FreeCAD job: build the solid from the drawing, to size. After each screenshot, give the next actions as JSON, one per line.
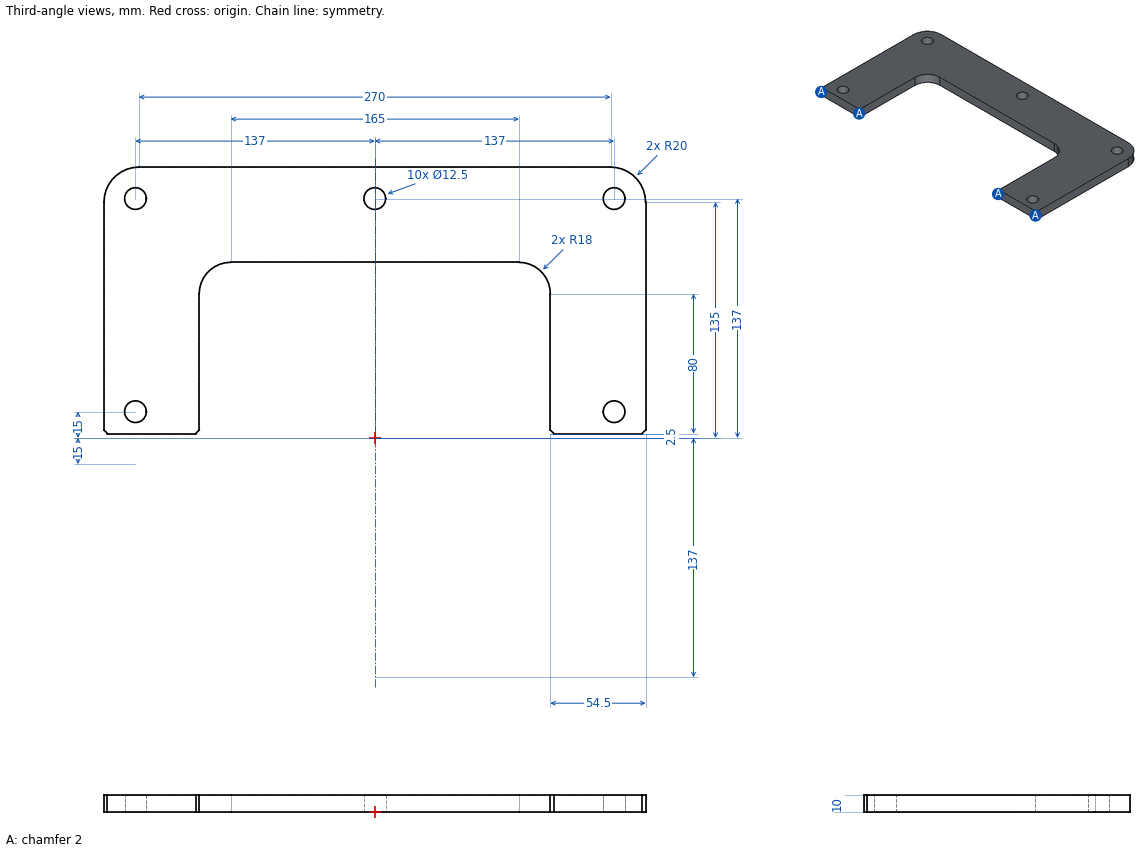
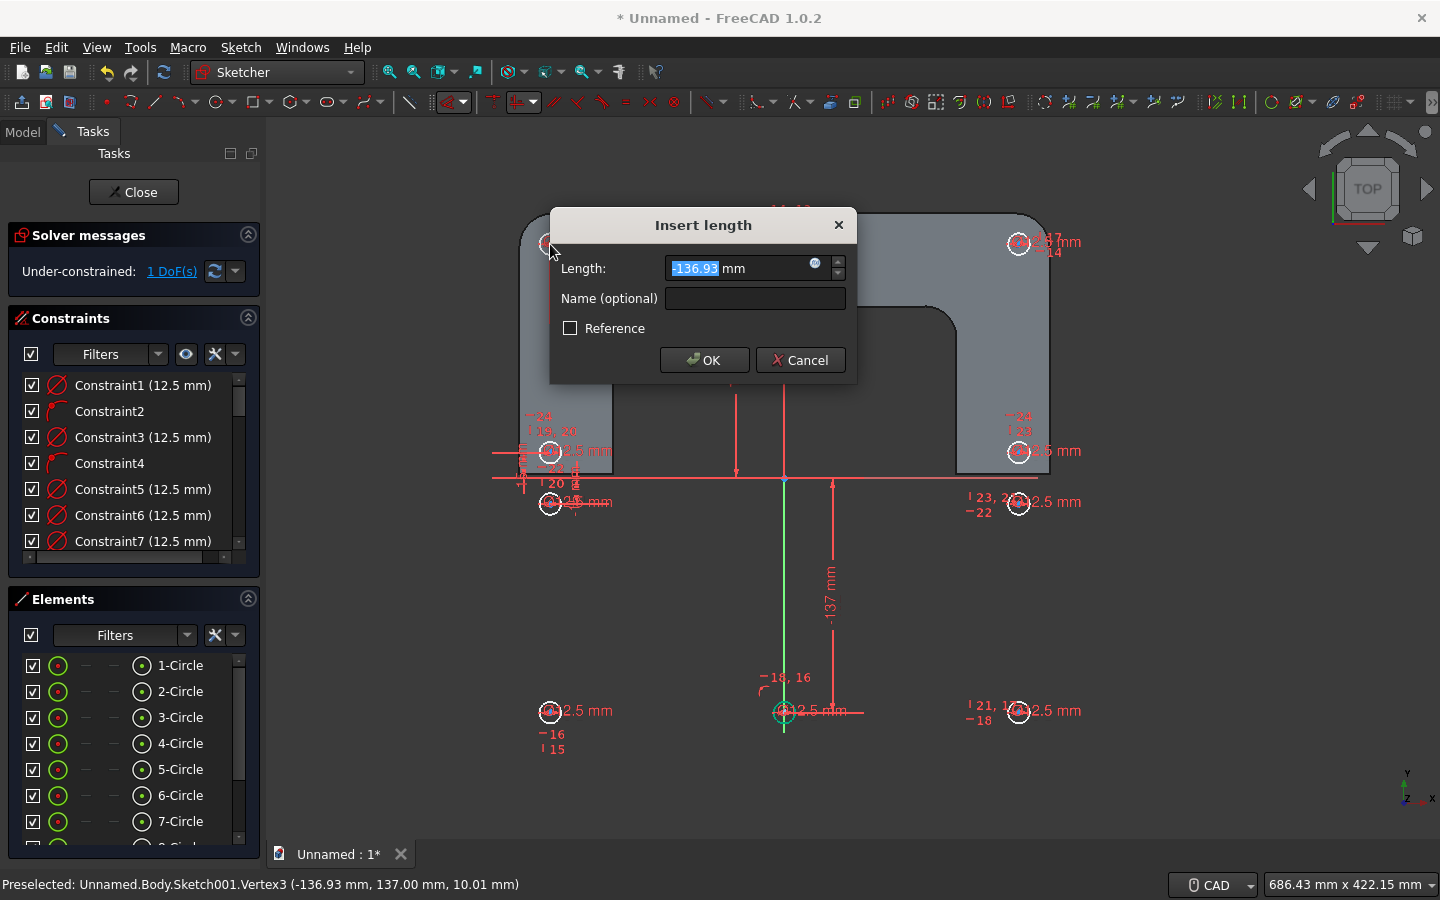
{"action": "type", "text": "-137"}
{"action": "key", "text": "Return"}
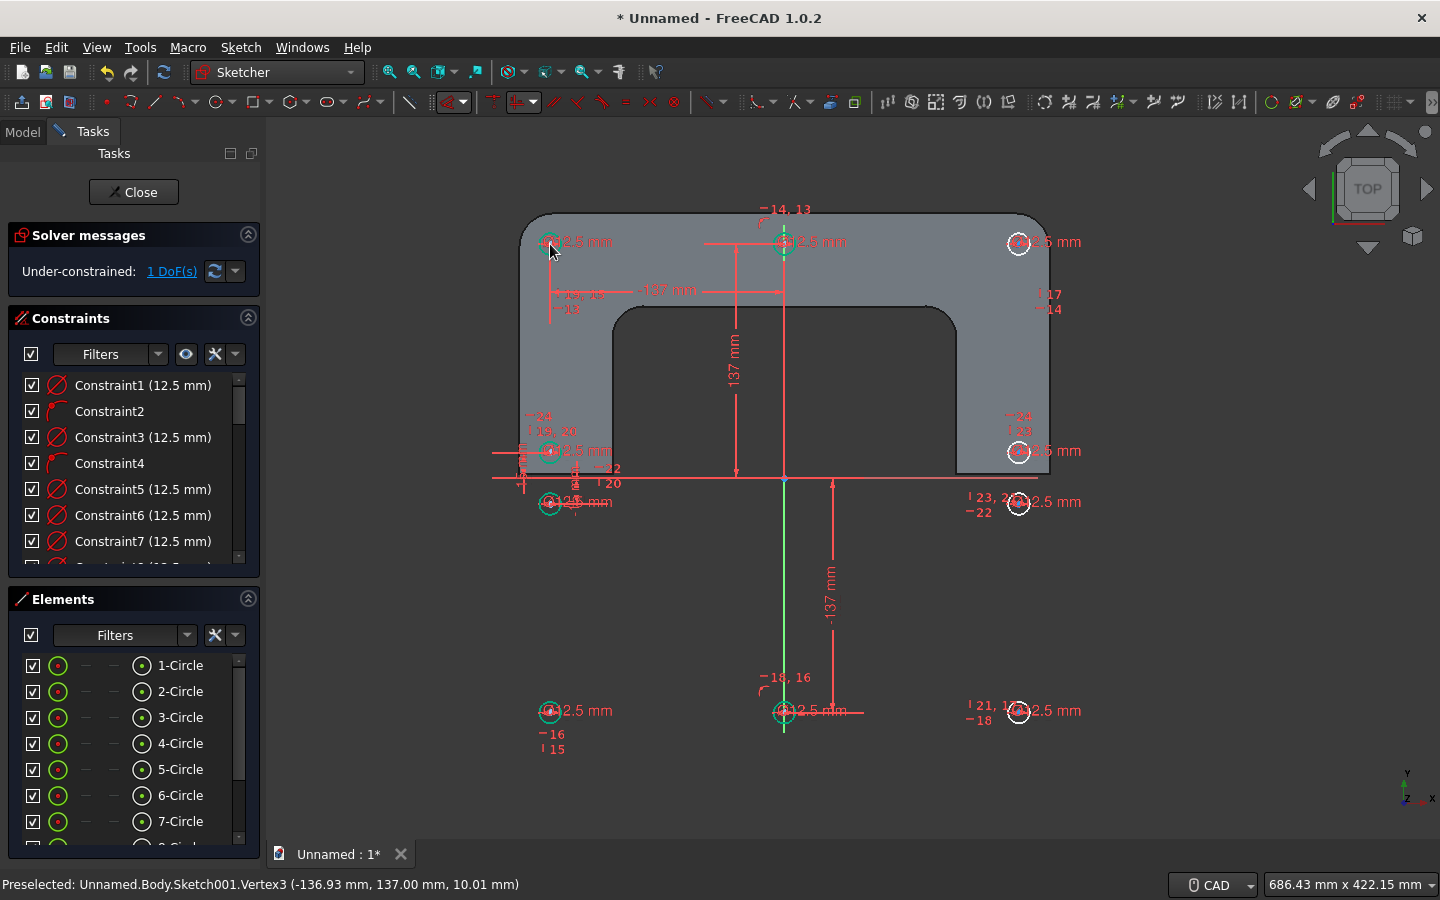
{"action": "left_click", "coordinate": [1019, 244]}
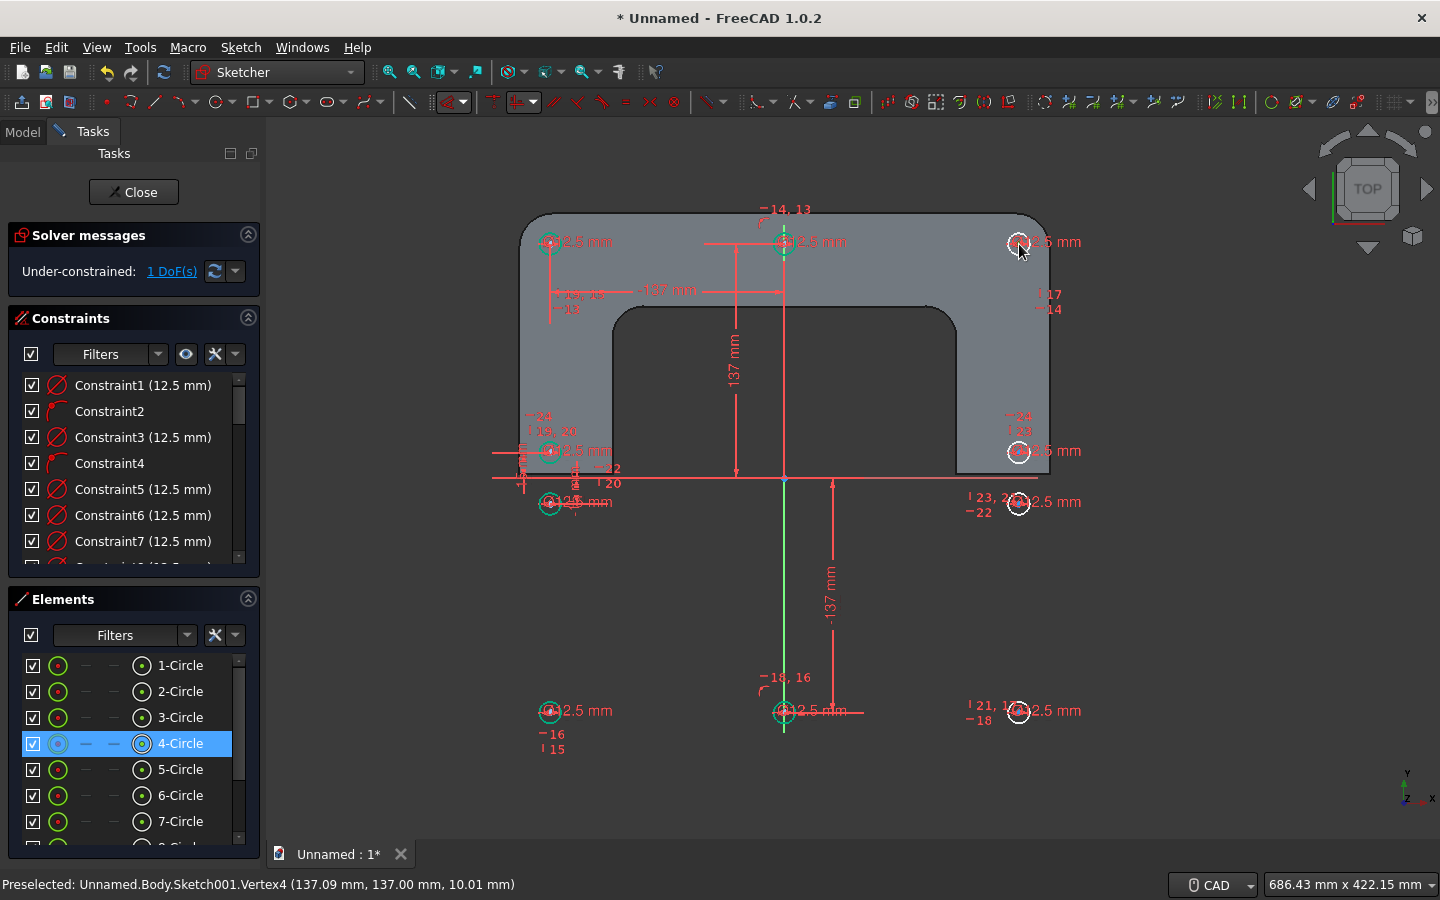
{"action": "key", "text": "l"}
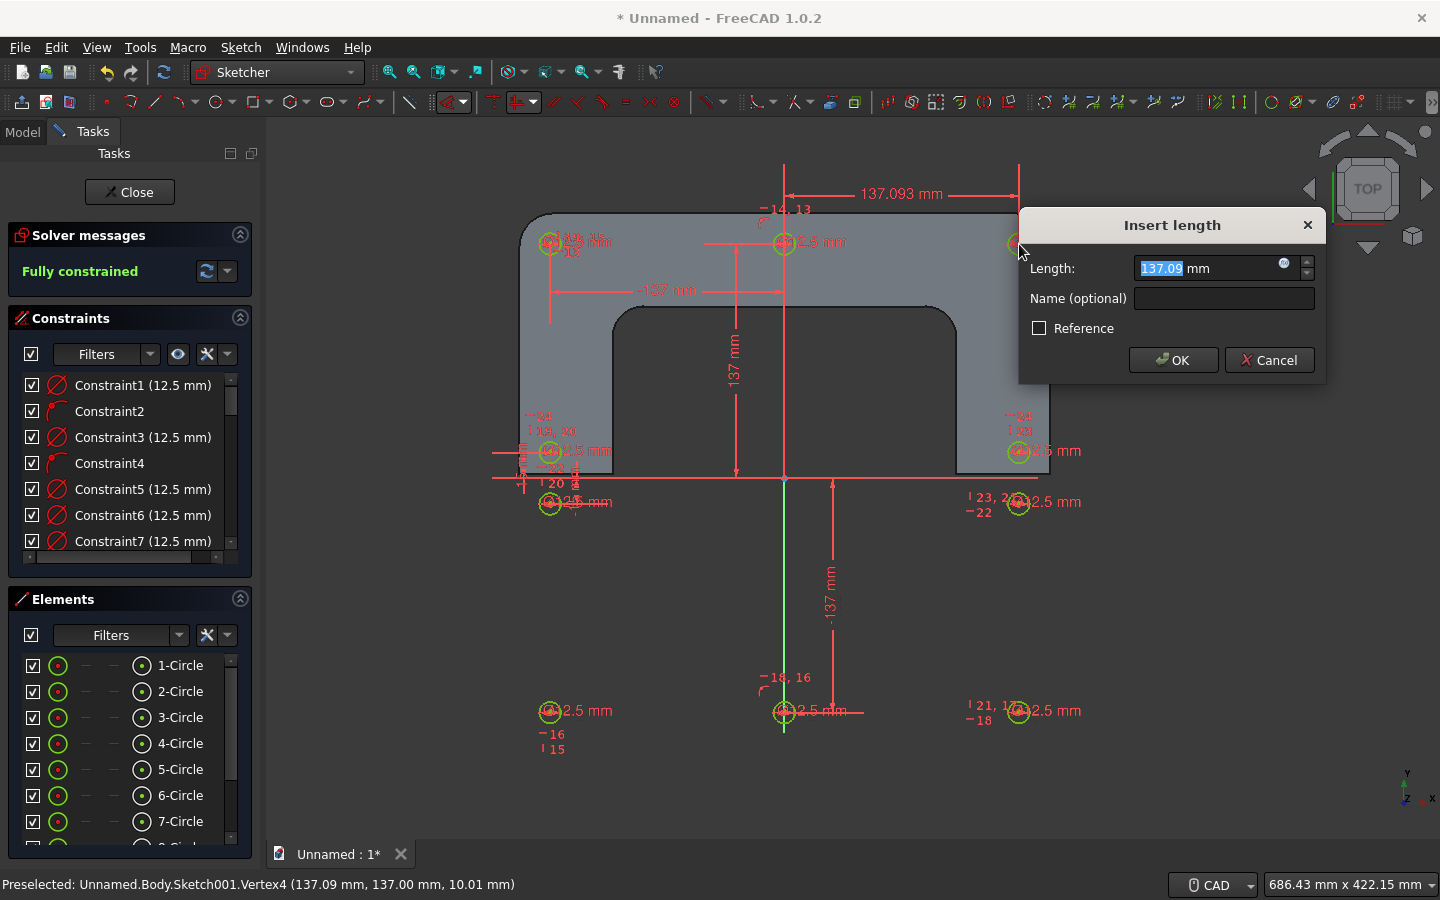
{"action": "type", "text": "137"}
{"action": "key", "text": "Return"}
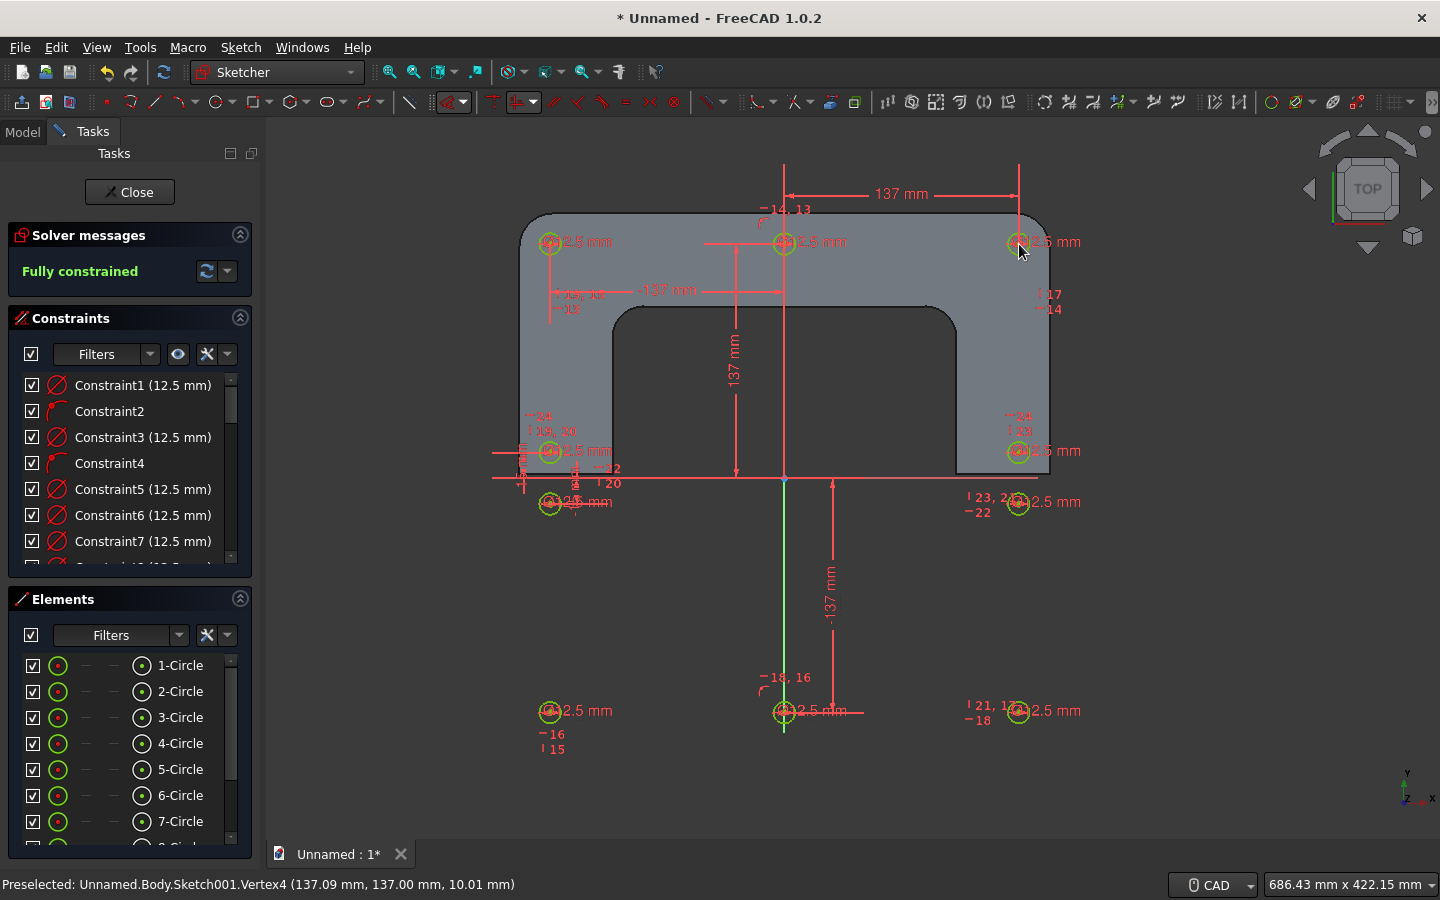
{"action": "left_click", "coordinate": [130, 192]}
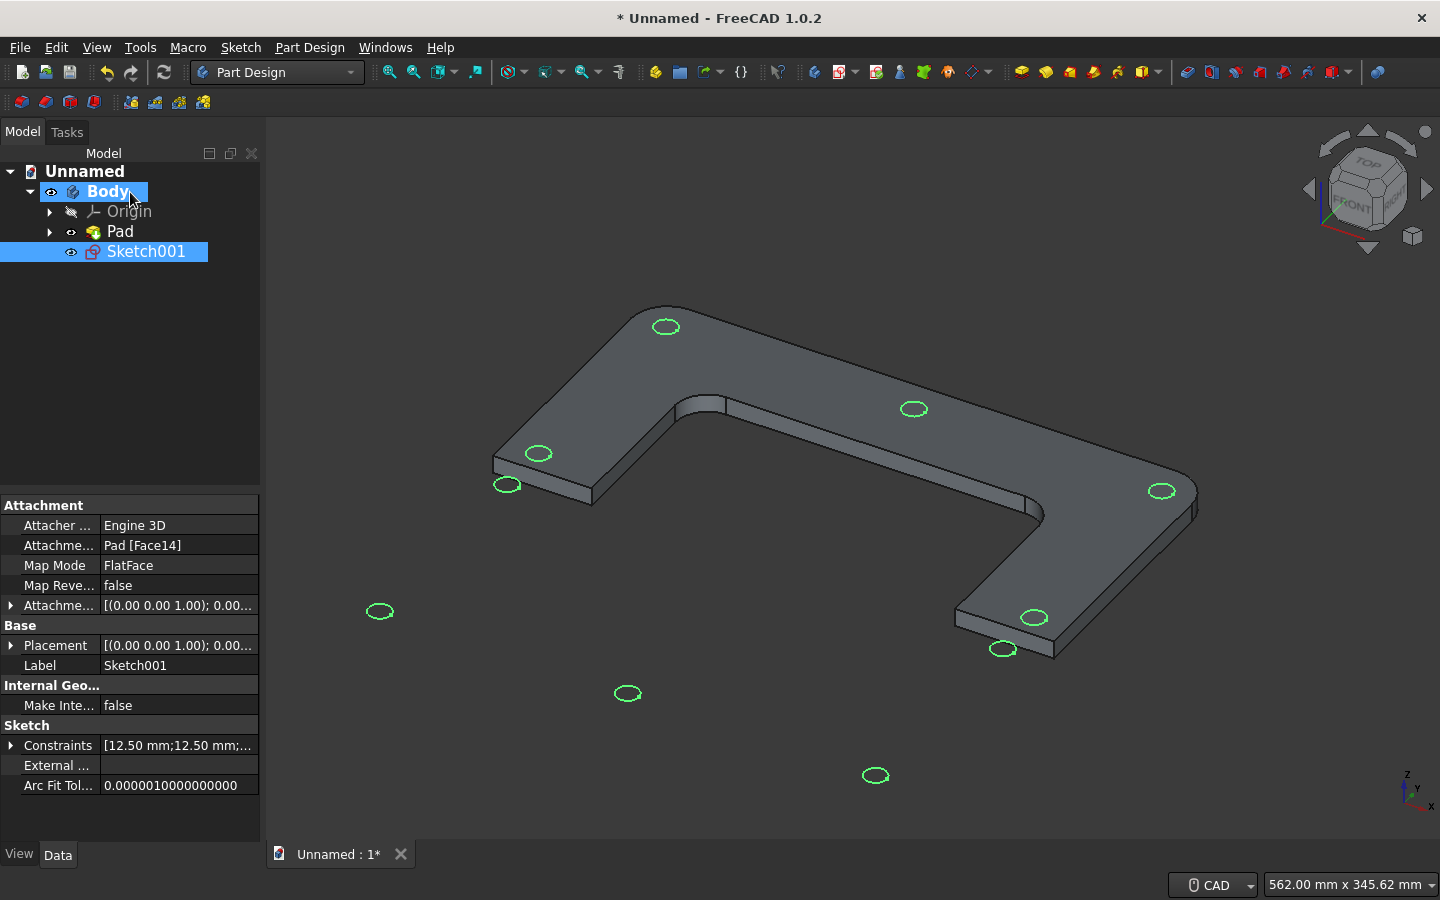
{"action": "left_click", "coordinate": [1188, 72]}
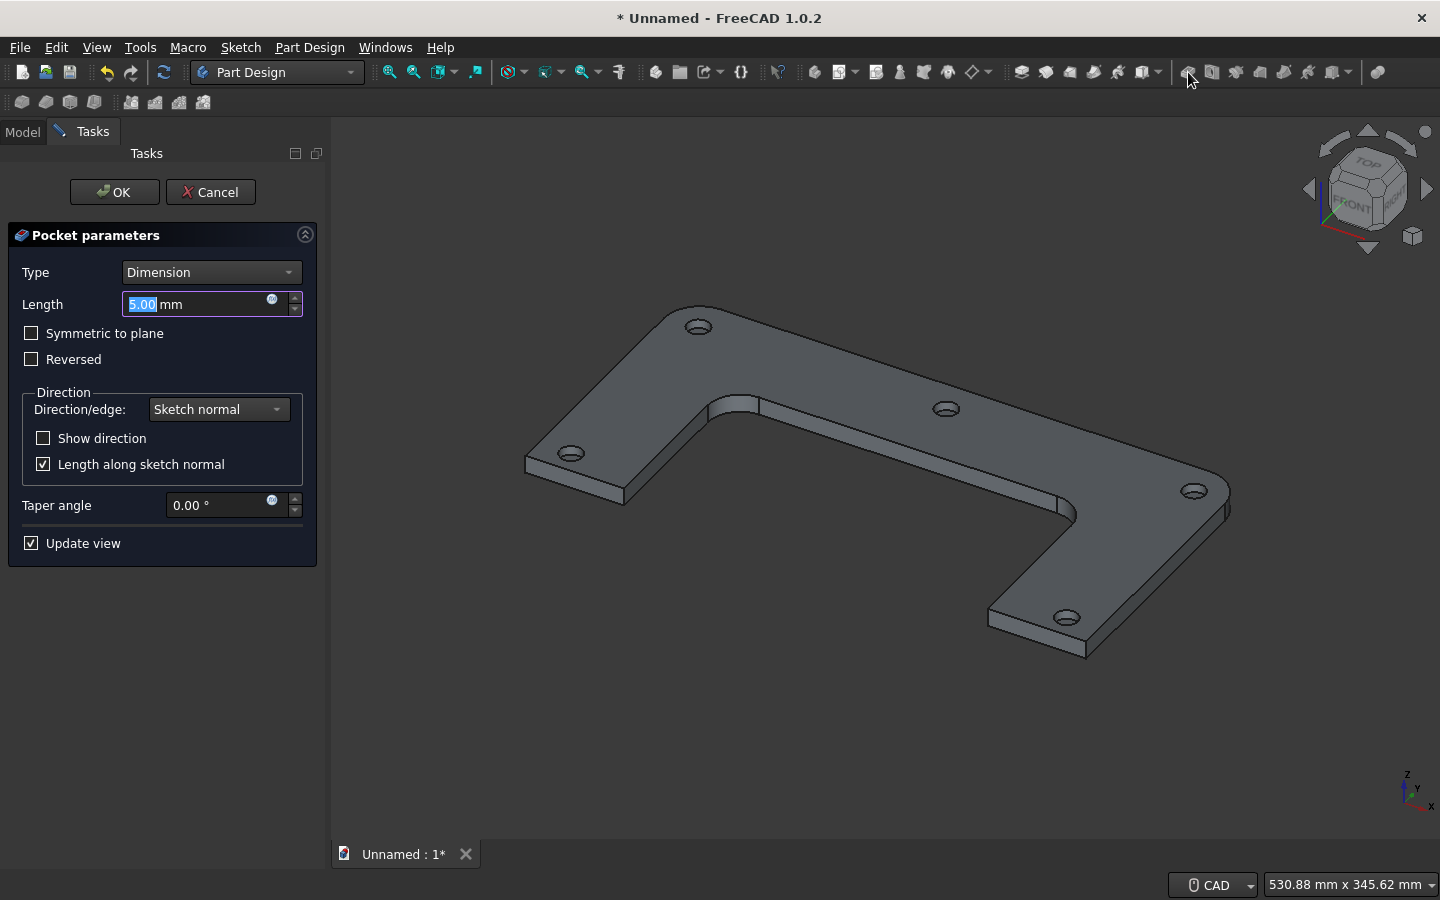
{"action": "left_click", "coordinate": [212, 272]}